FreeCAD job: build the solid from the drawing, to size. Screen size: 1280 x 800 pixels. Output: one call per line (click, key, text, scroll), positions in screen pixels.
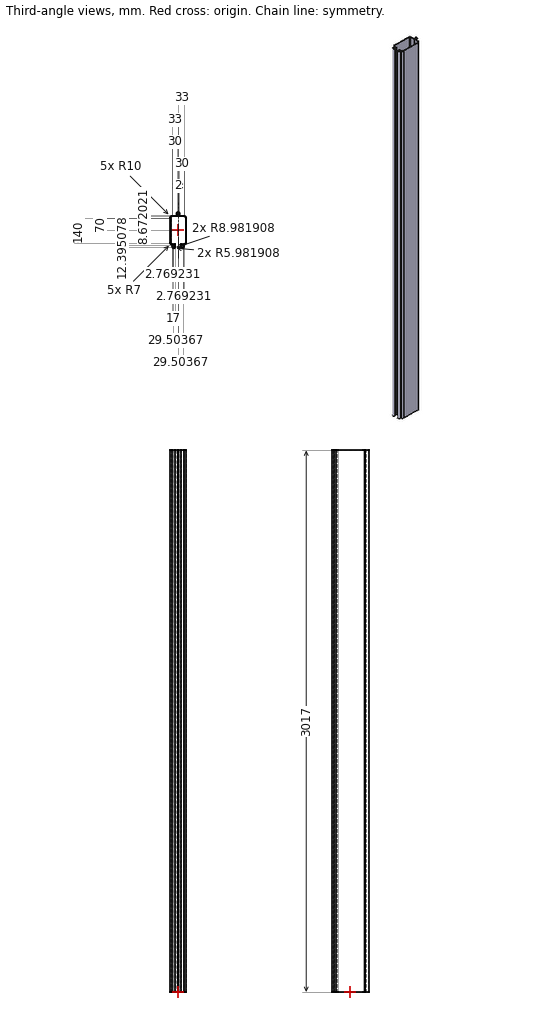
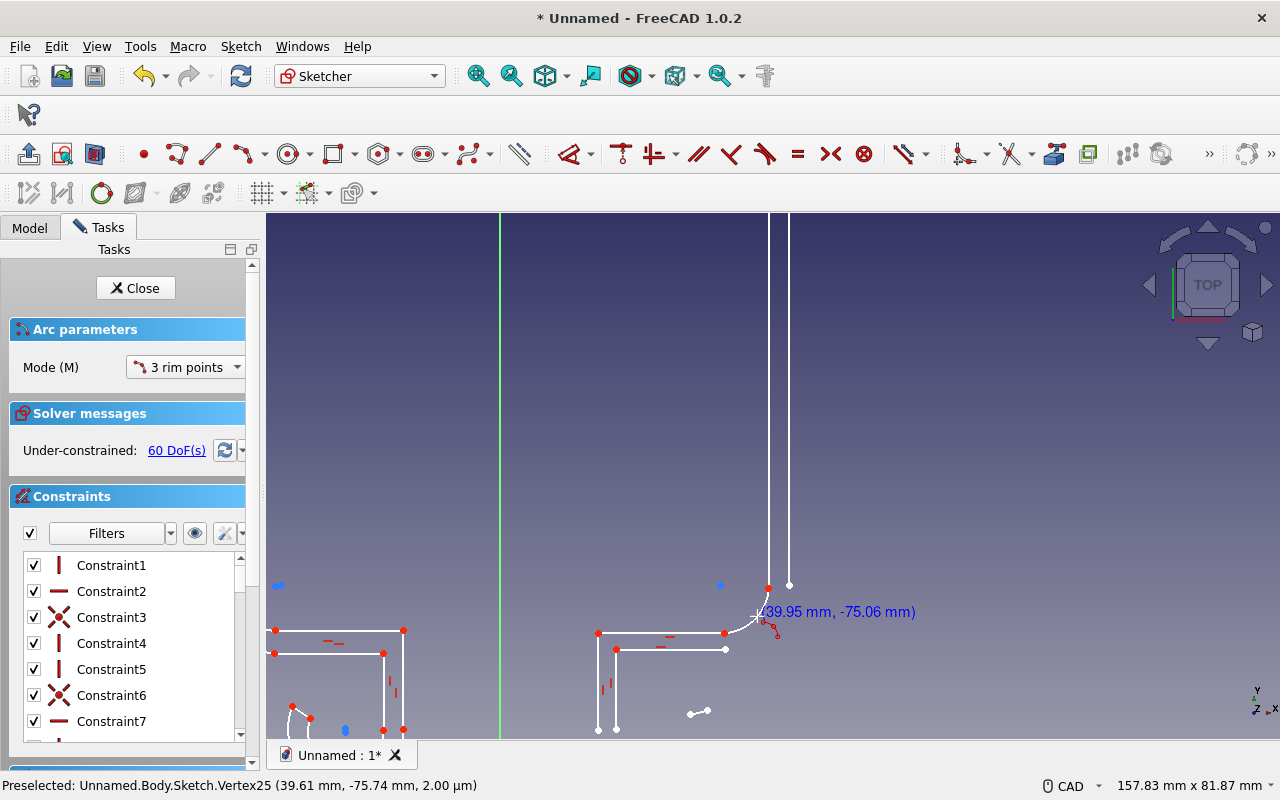
scroll(771, 589, down, 7)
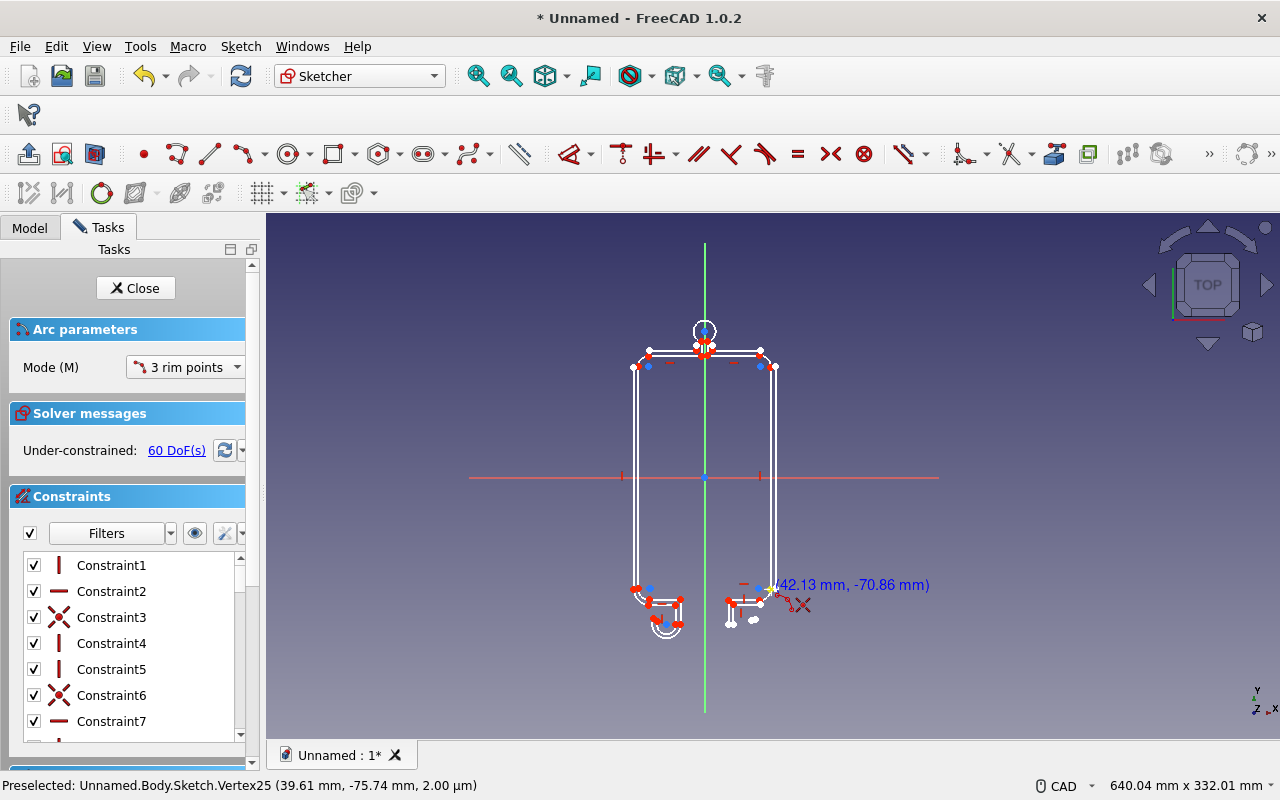
scroll(728, 624, up, 7)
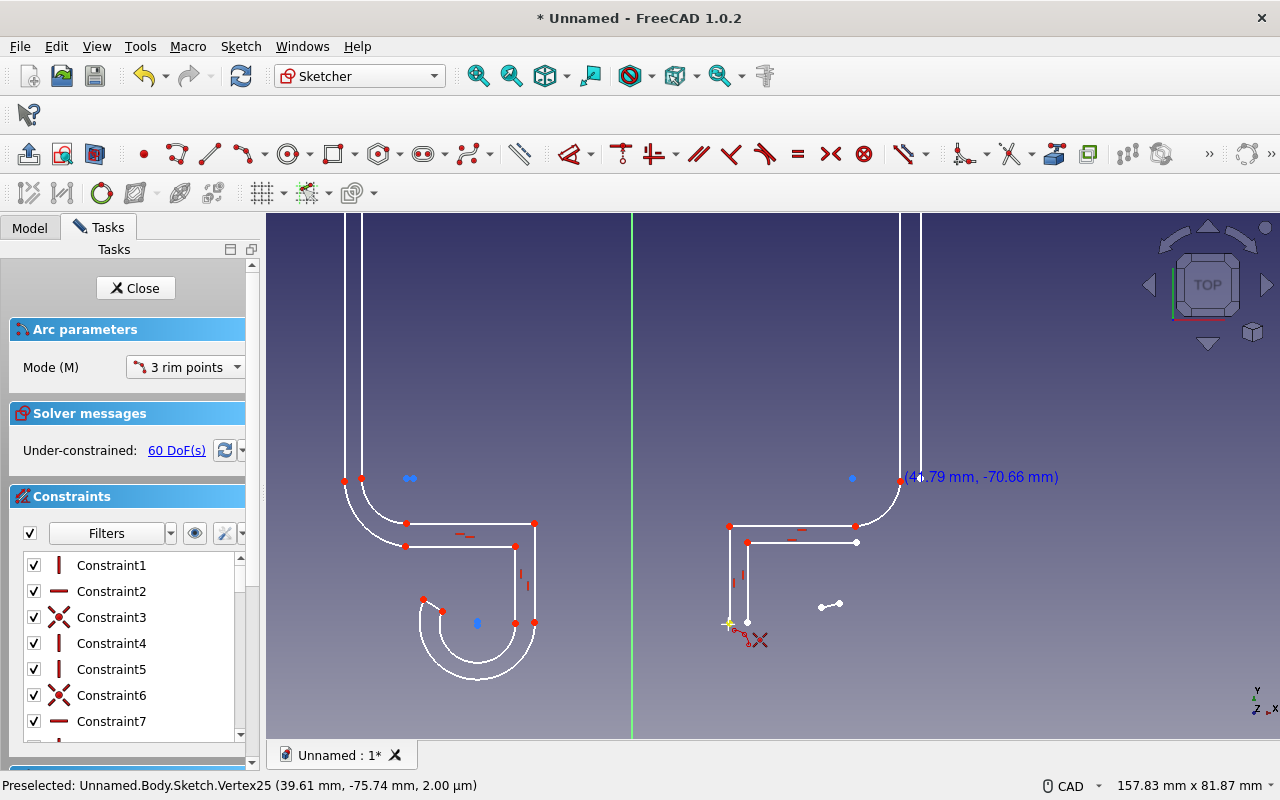
click(730, 624)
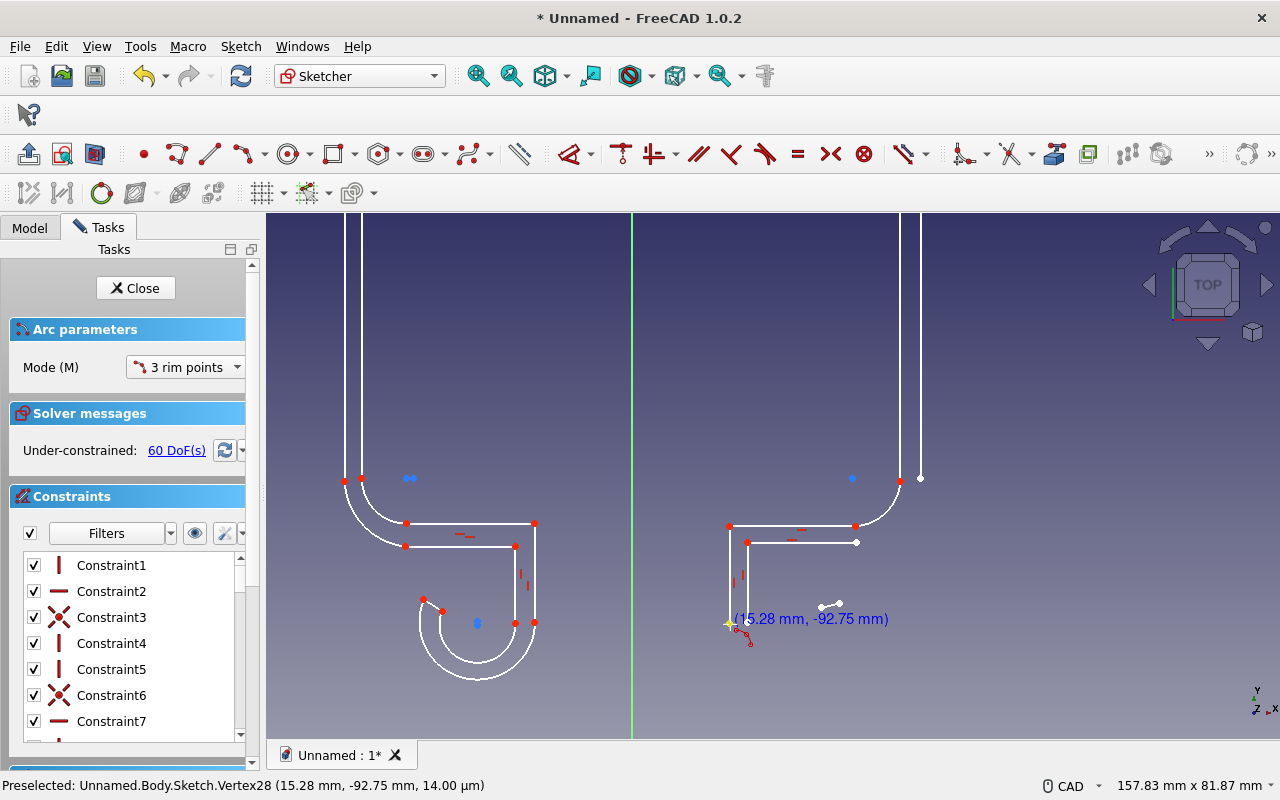
scroll(839, 599, up, 3)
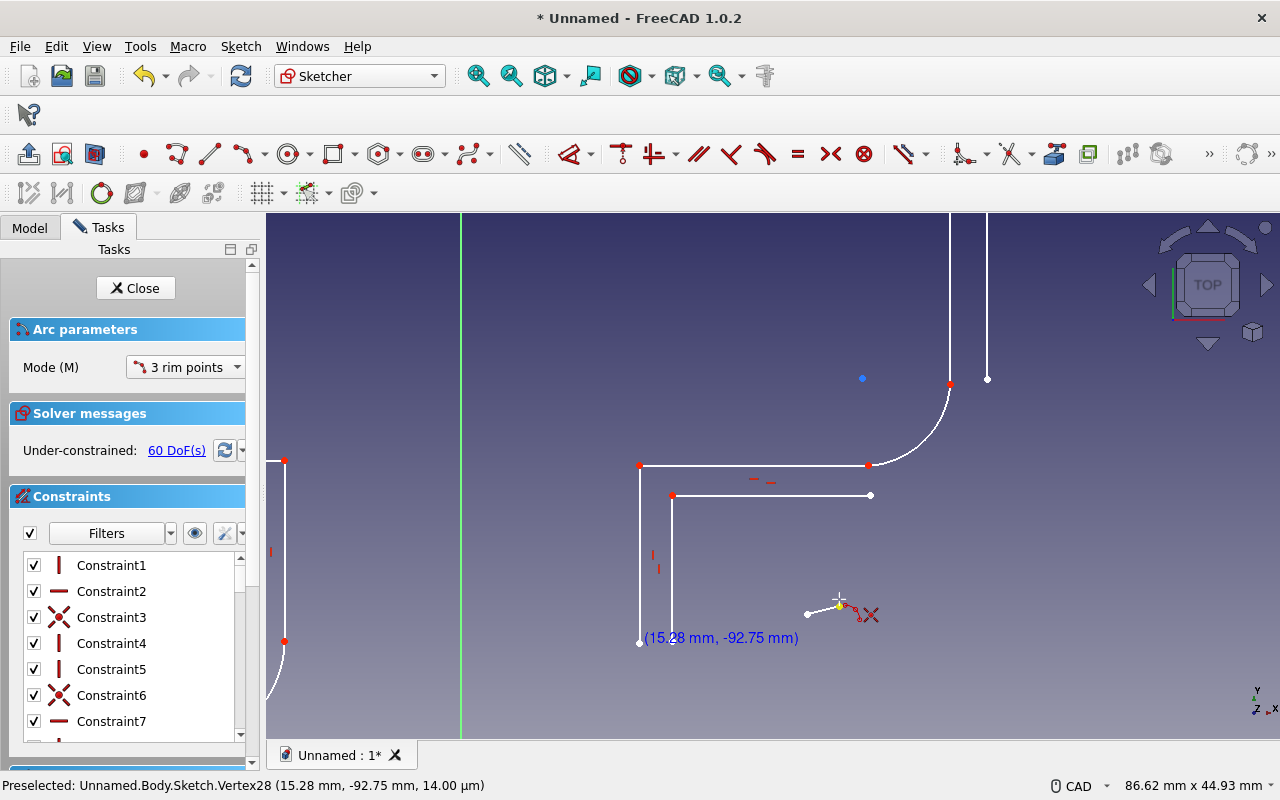
click(839, 606)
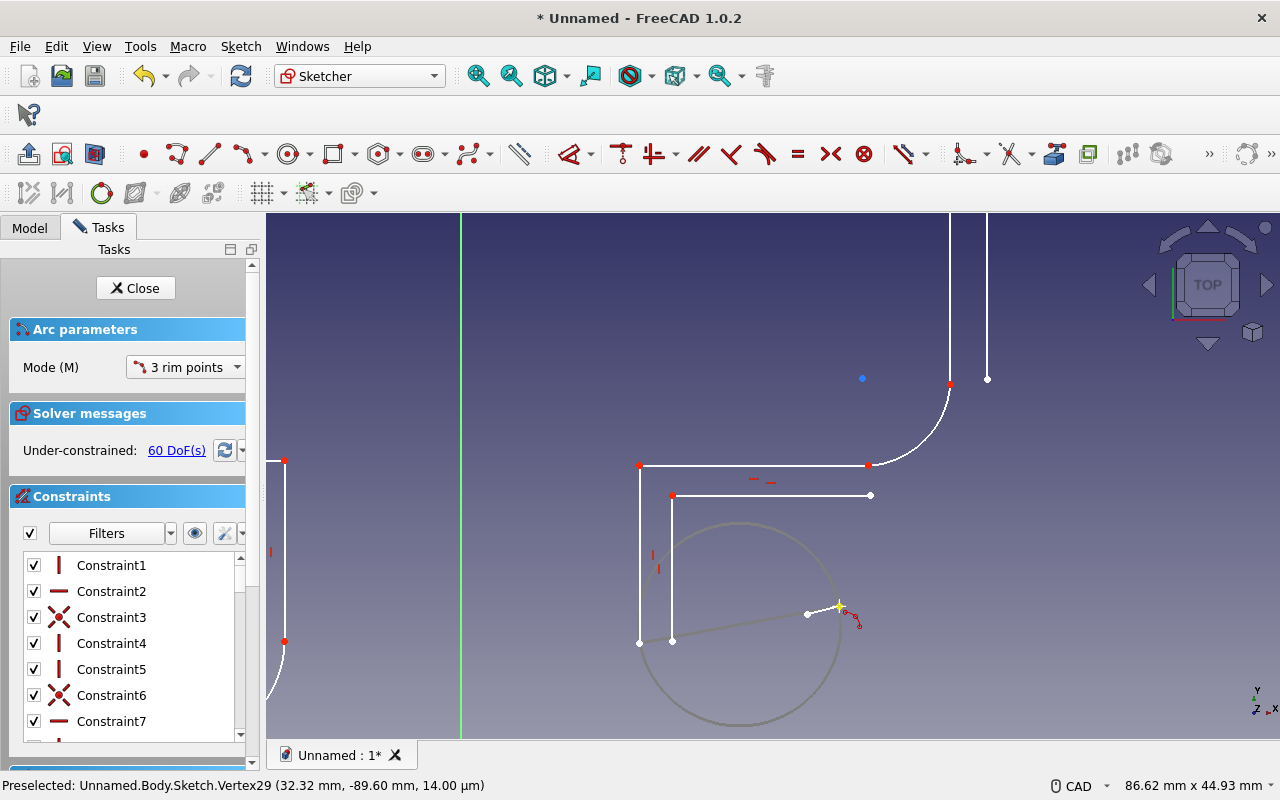
scroll(743, 621, down, 10)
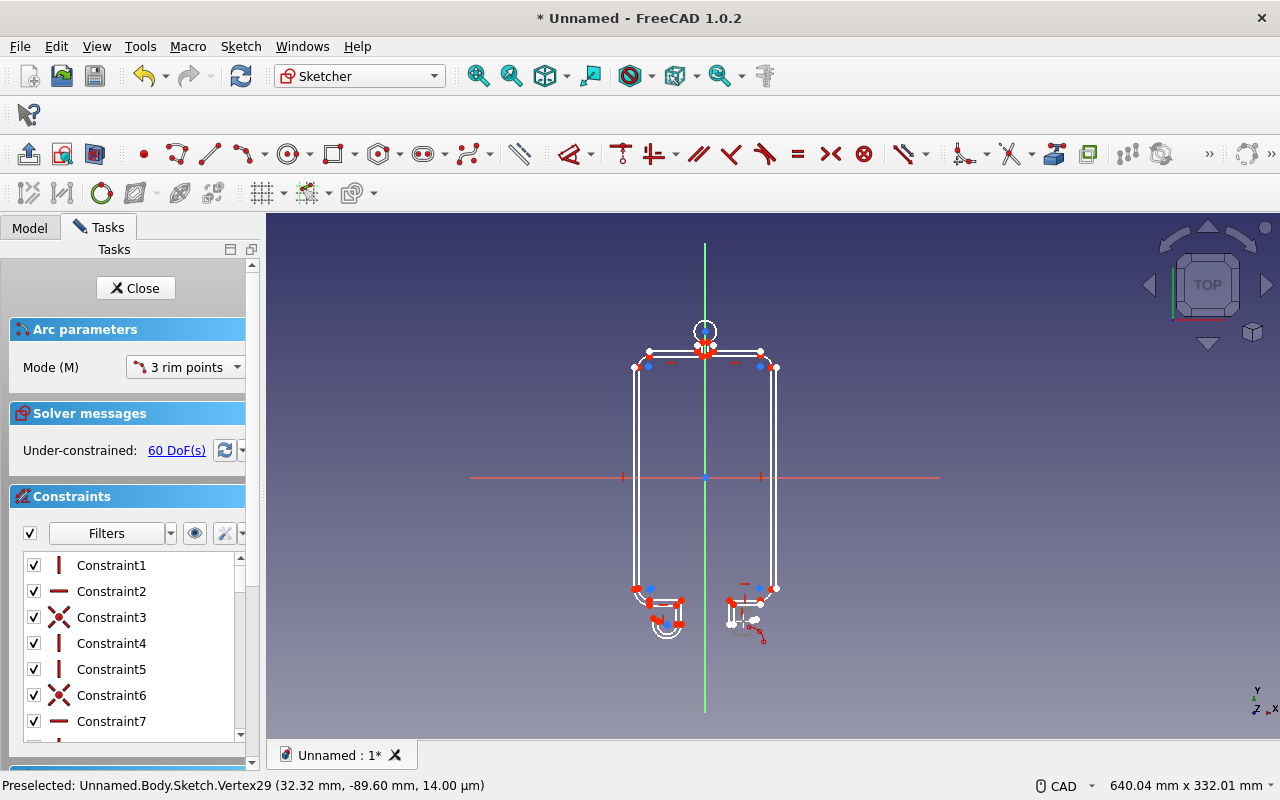
click(746, 638)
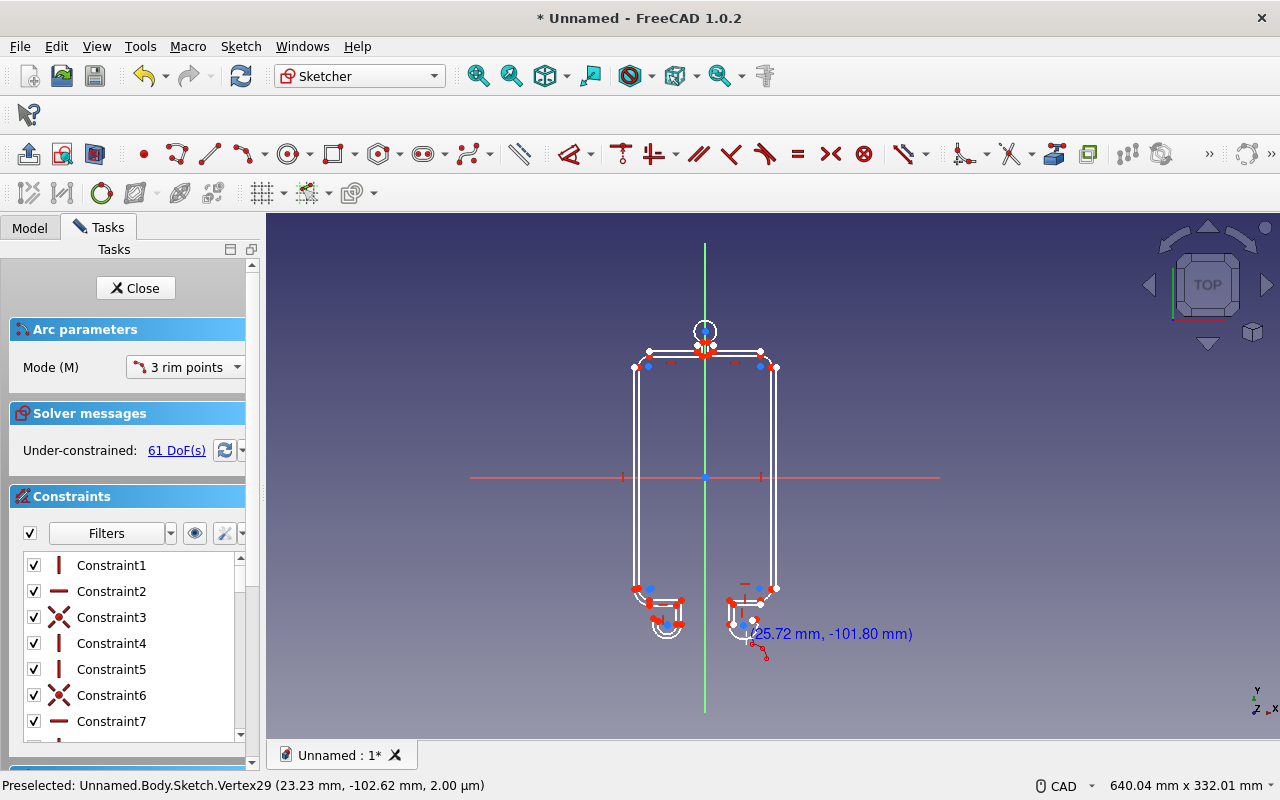
scroll(752, 620, up, 10)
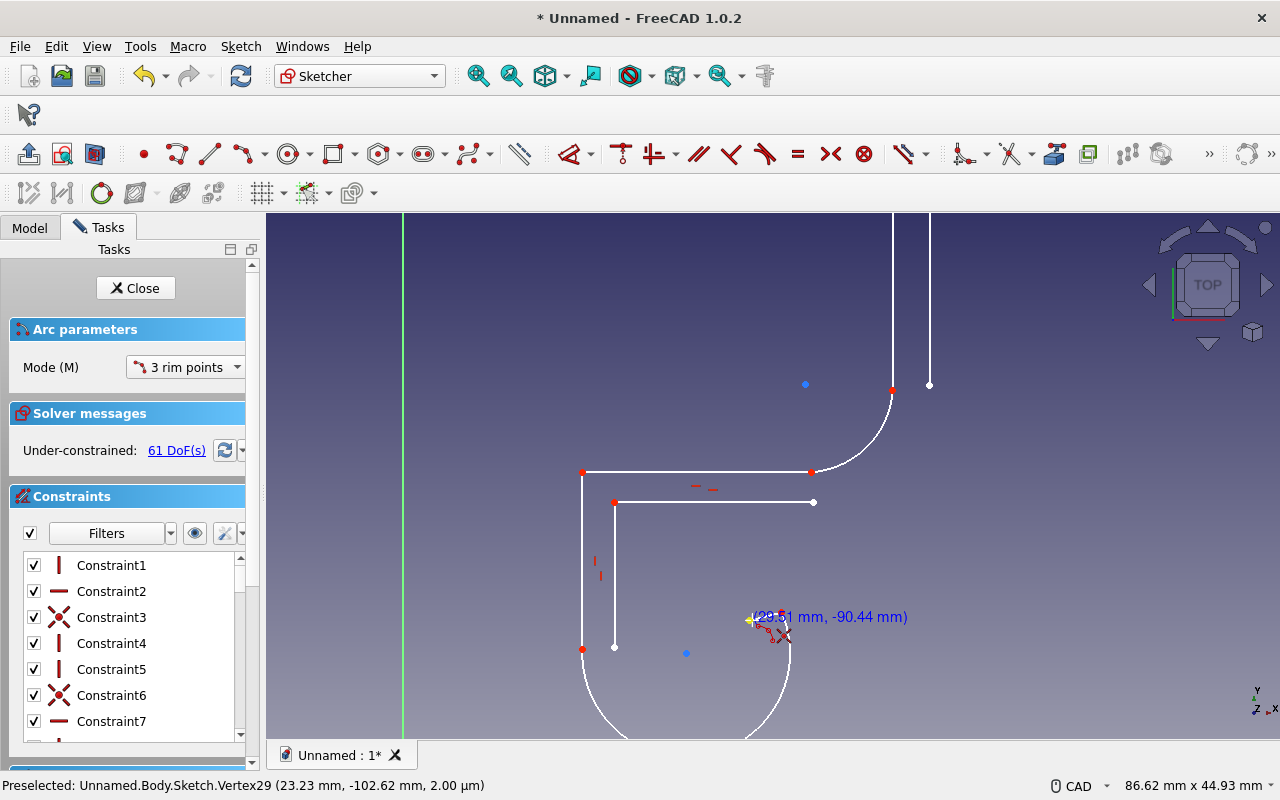
click(749, 621)
click(615, 648)
click(721, 705)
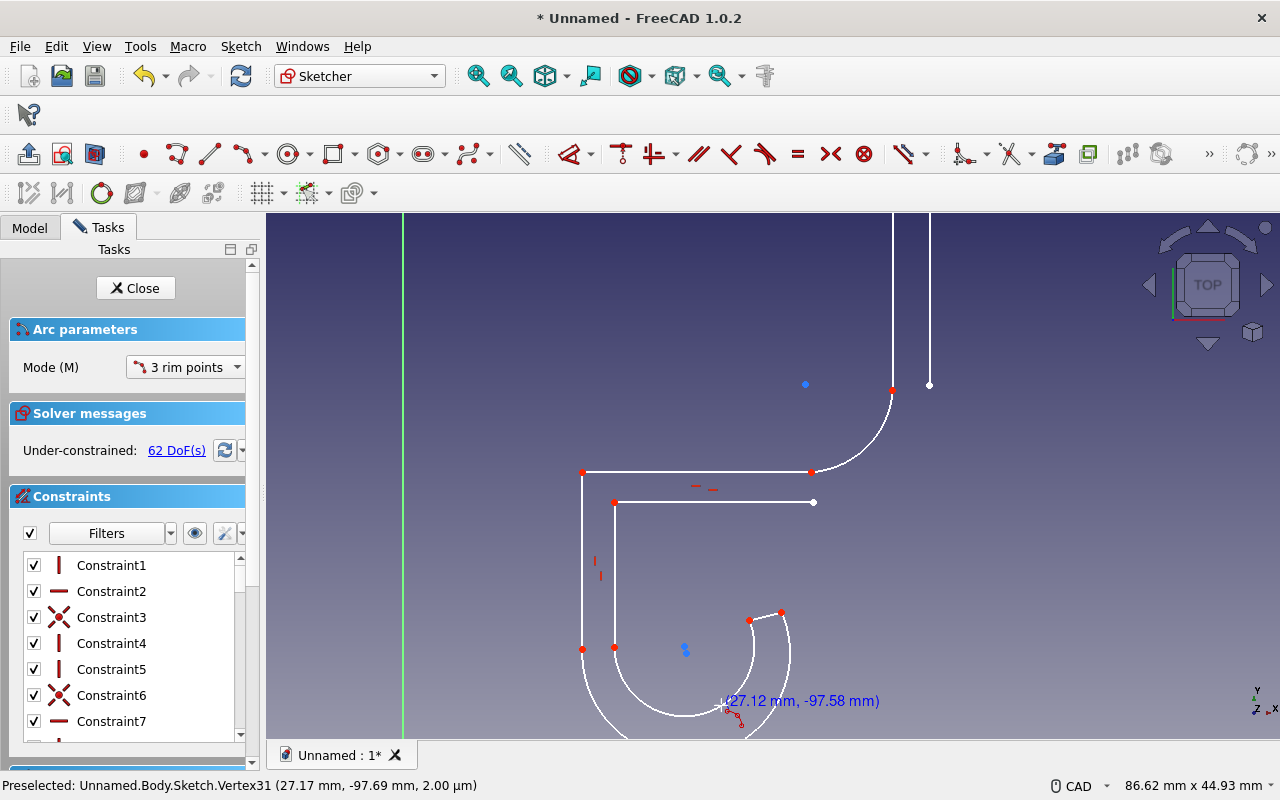
click(813, 502)
click(930, 386)
click(896, 466)